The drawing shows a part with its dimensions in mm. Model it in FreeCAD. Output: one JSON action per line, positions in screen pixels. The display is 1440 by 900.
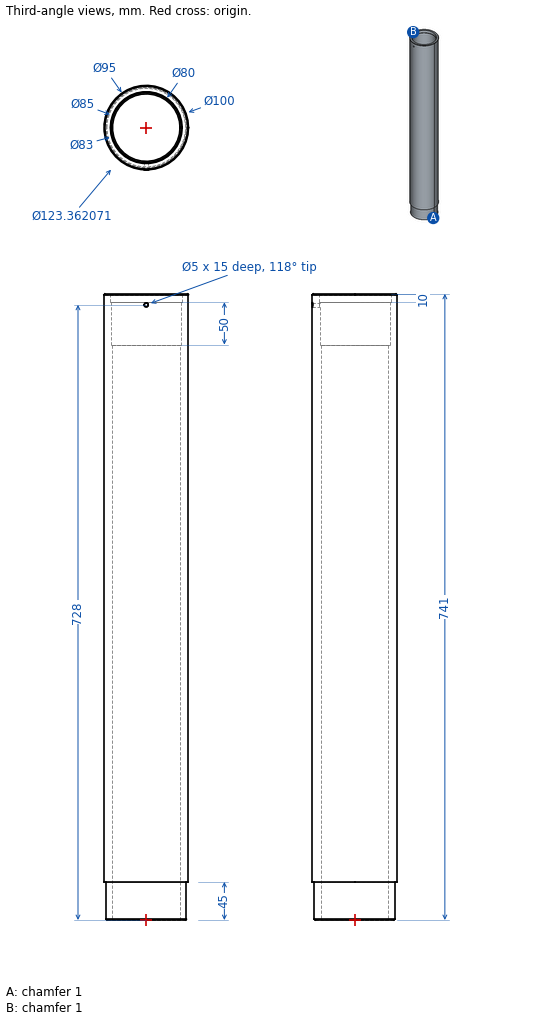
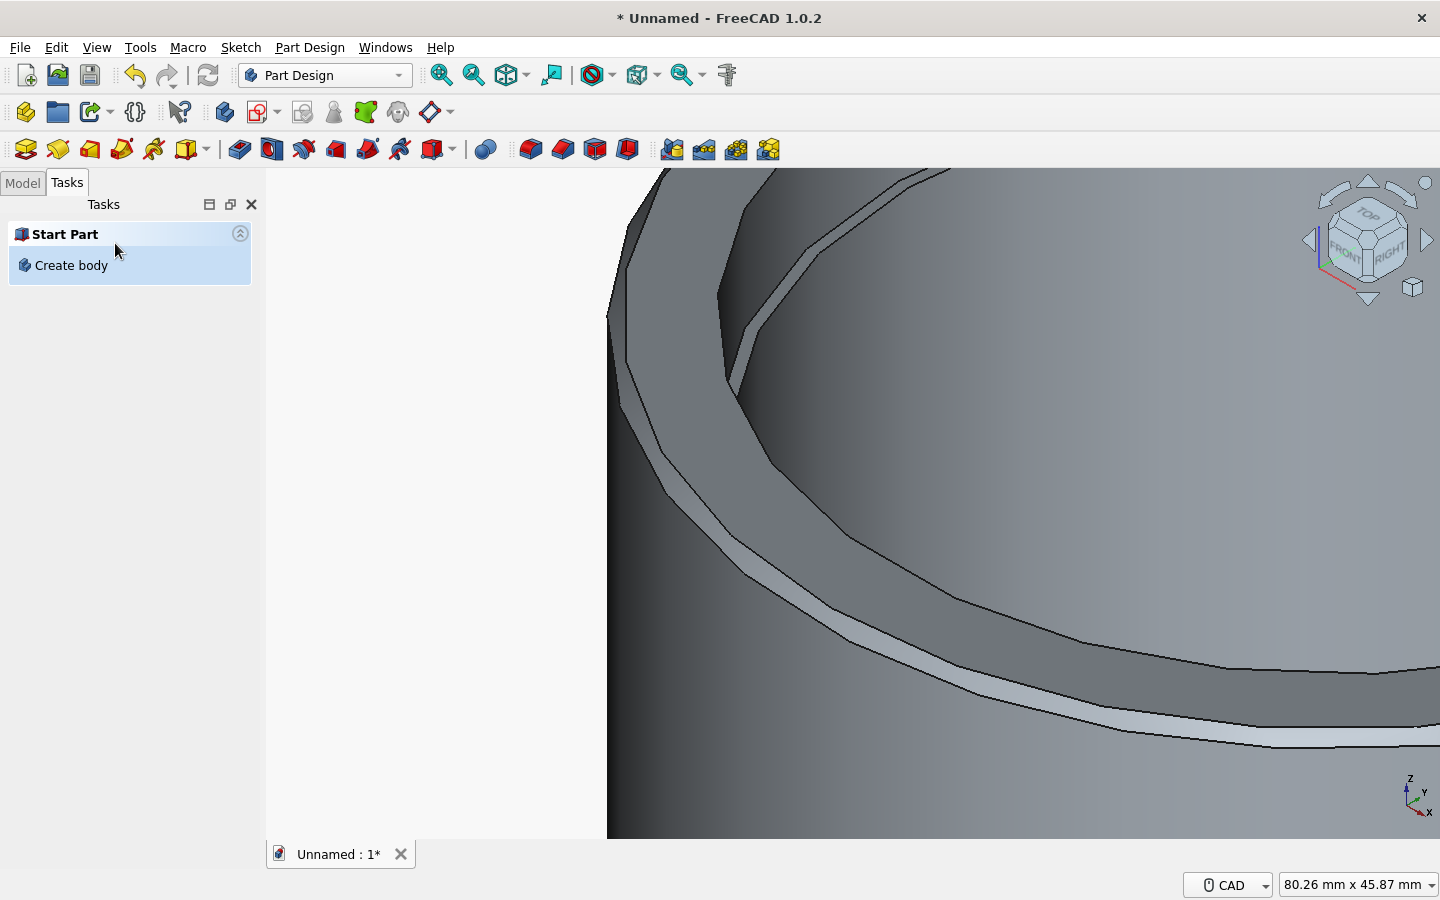
{"action": "left_click", "coordinate": [442, 76]}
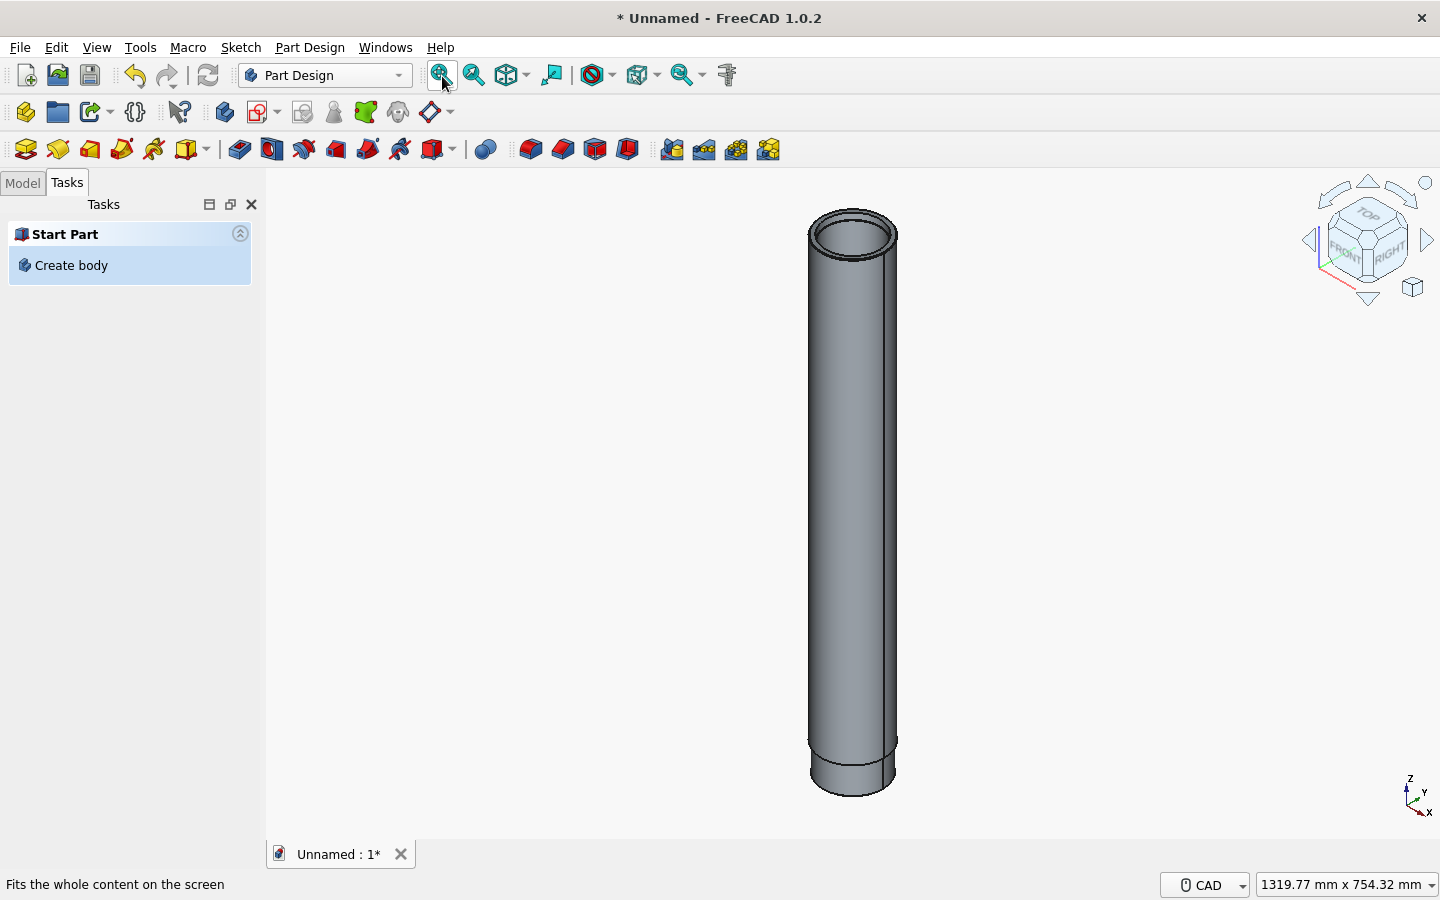
{"action": "left_click", "coordinate": [23, 182]}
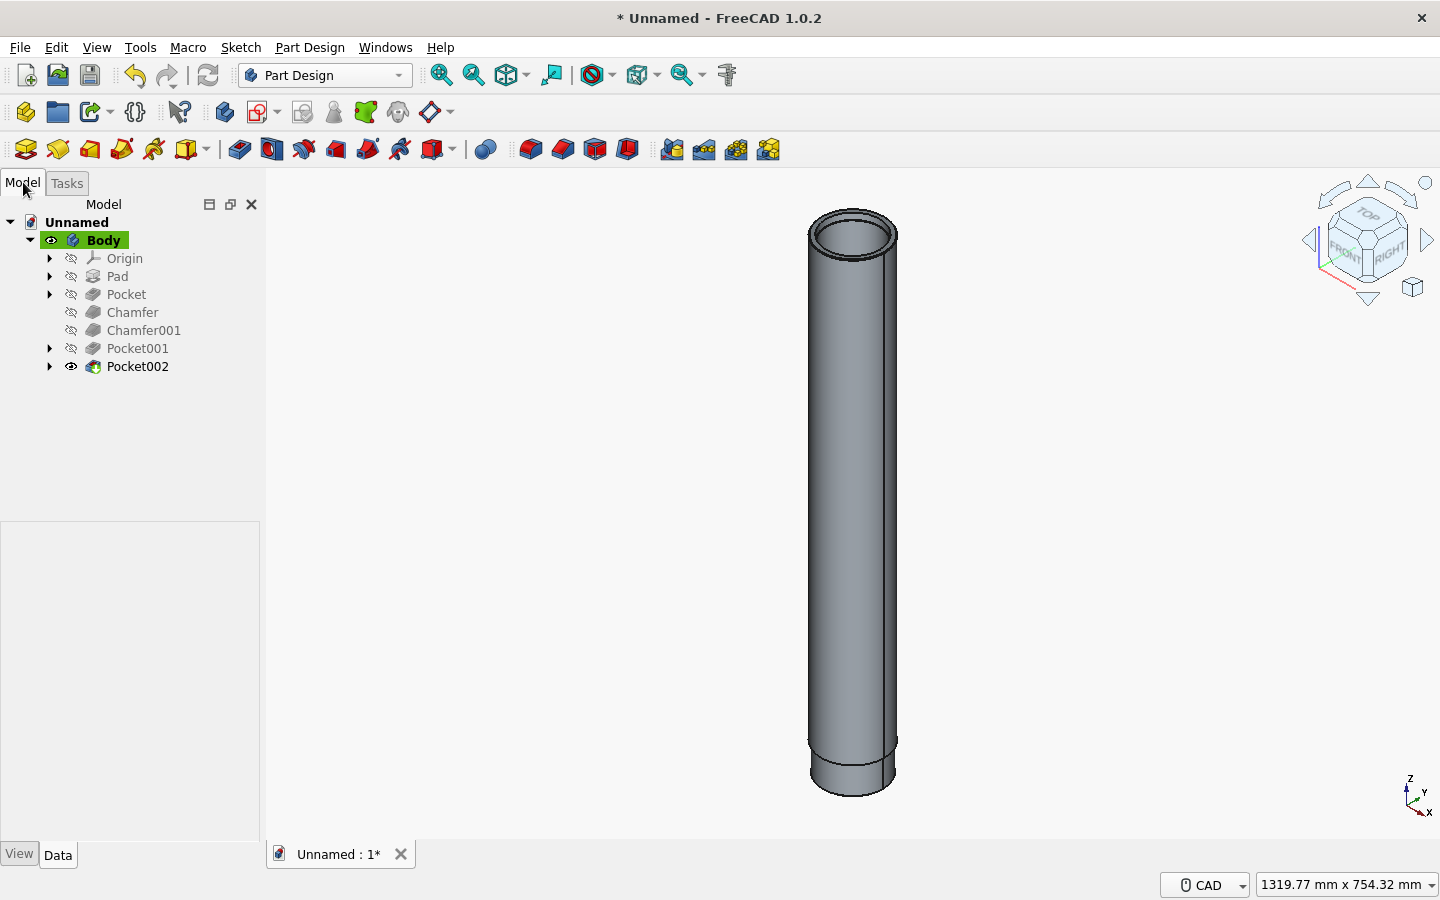
{"action": "left_click", "coordinate": [50, 258]}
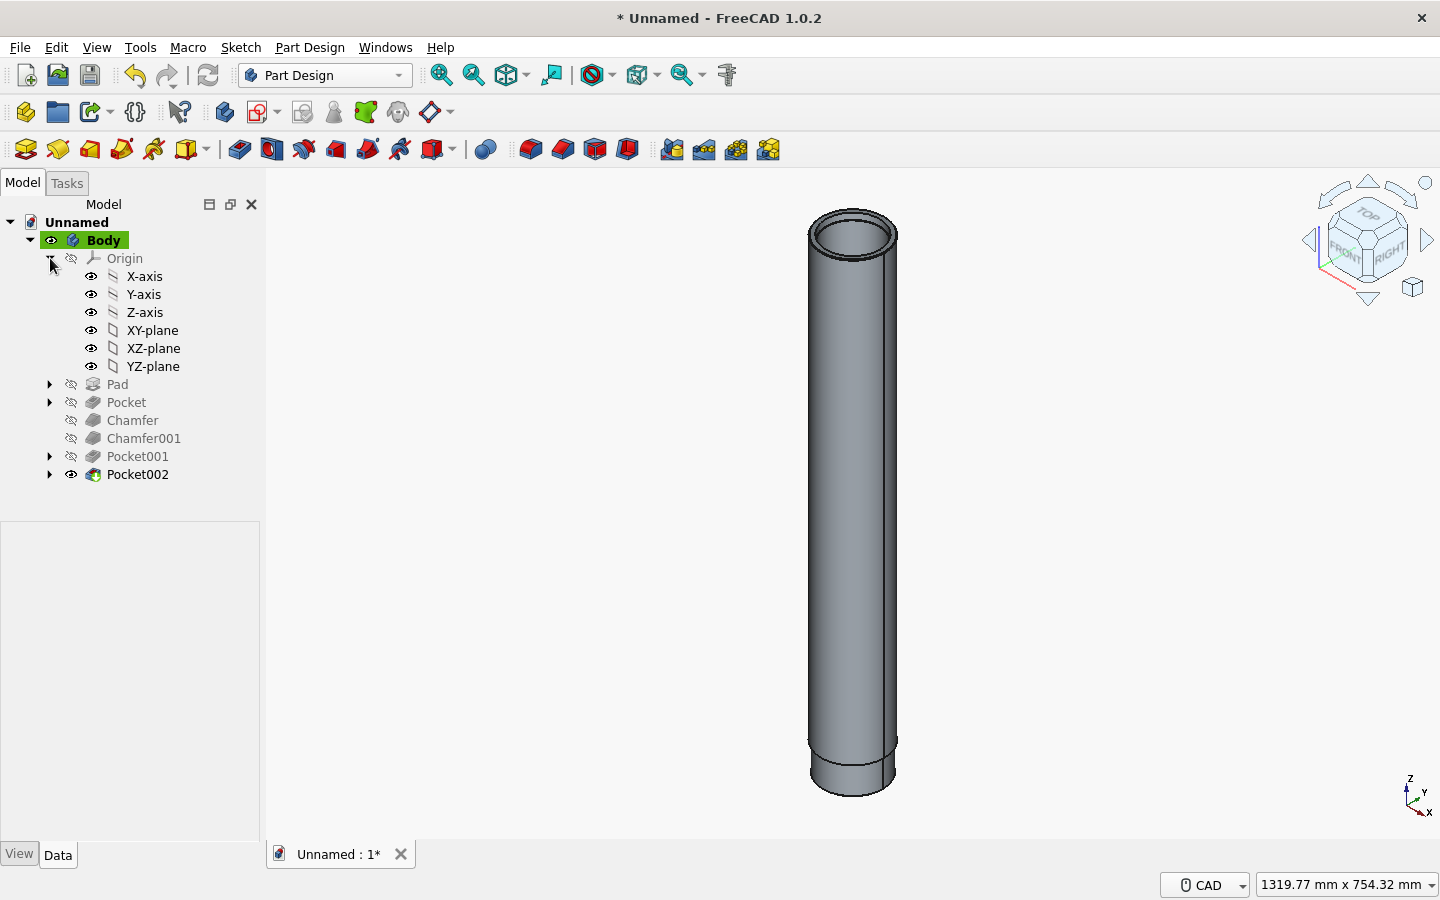
{"action": "left_click", "coordinate": [136, 348]}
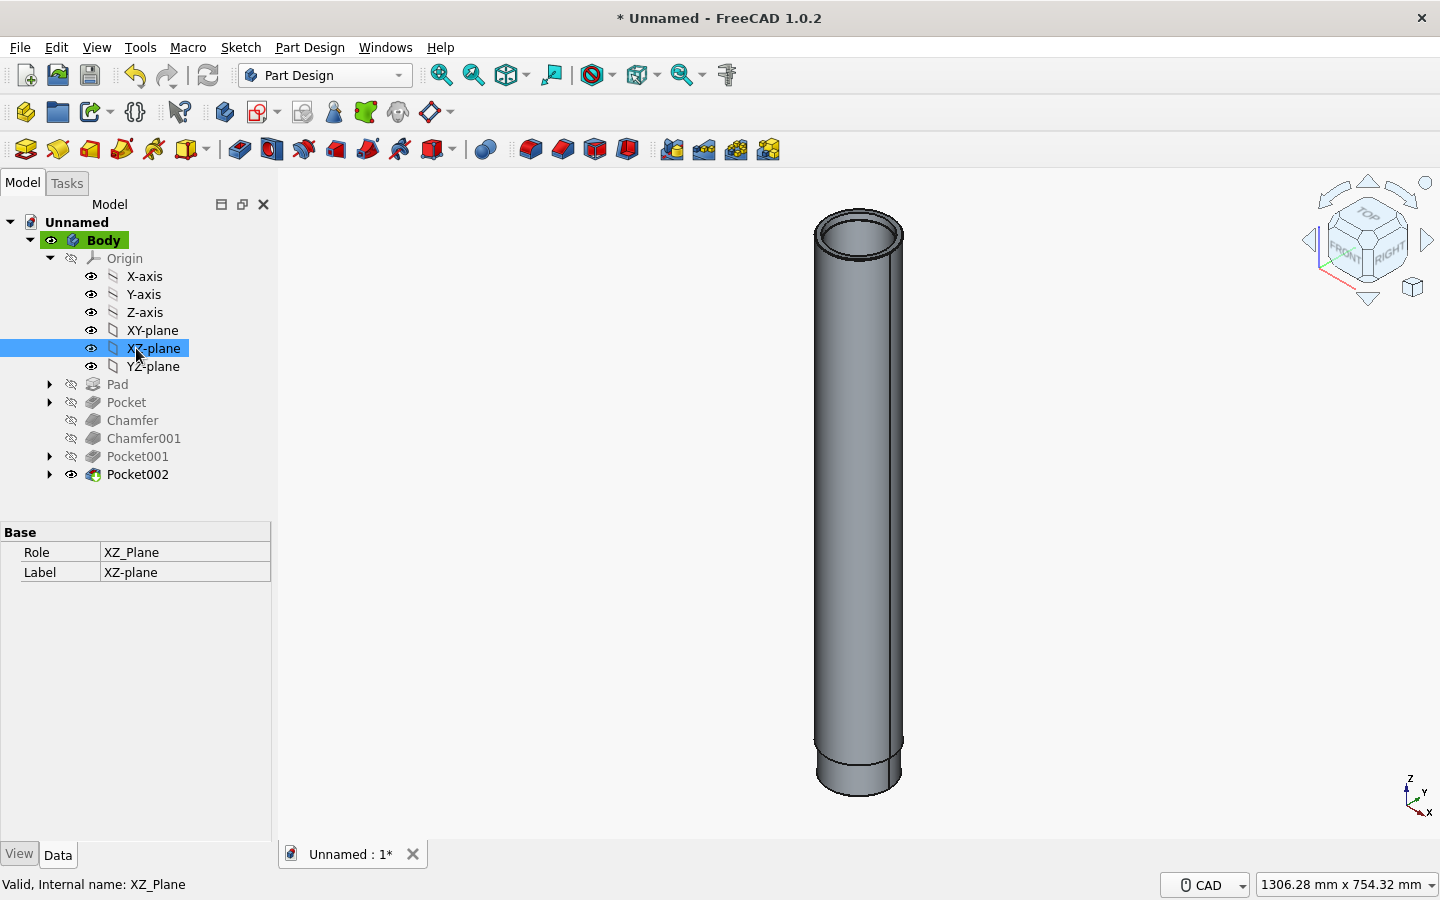
{"action": "left_click", "coordinate": [430, 112]}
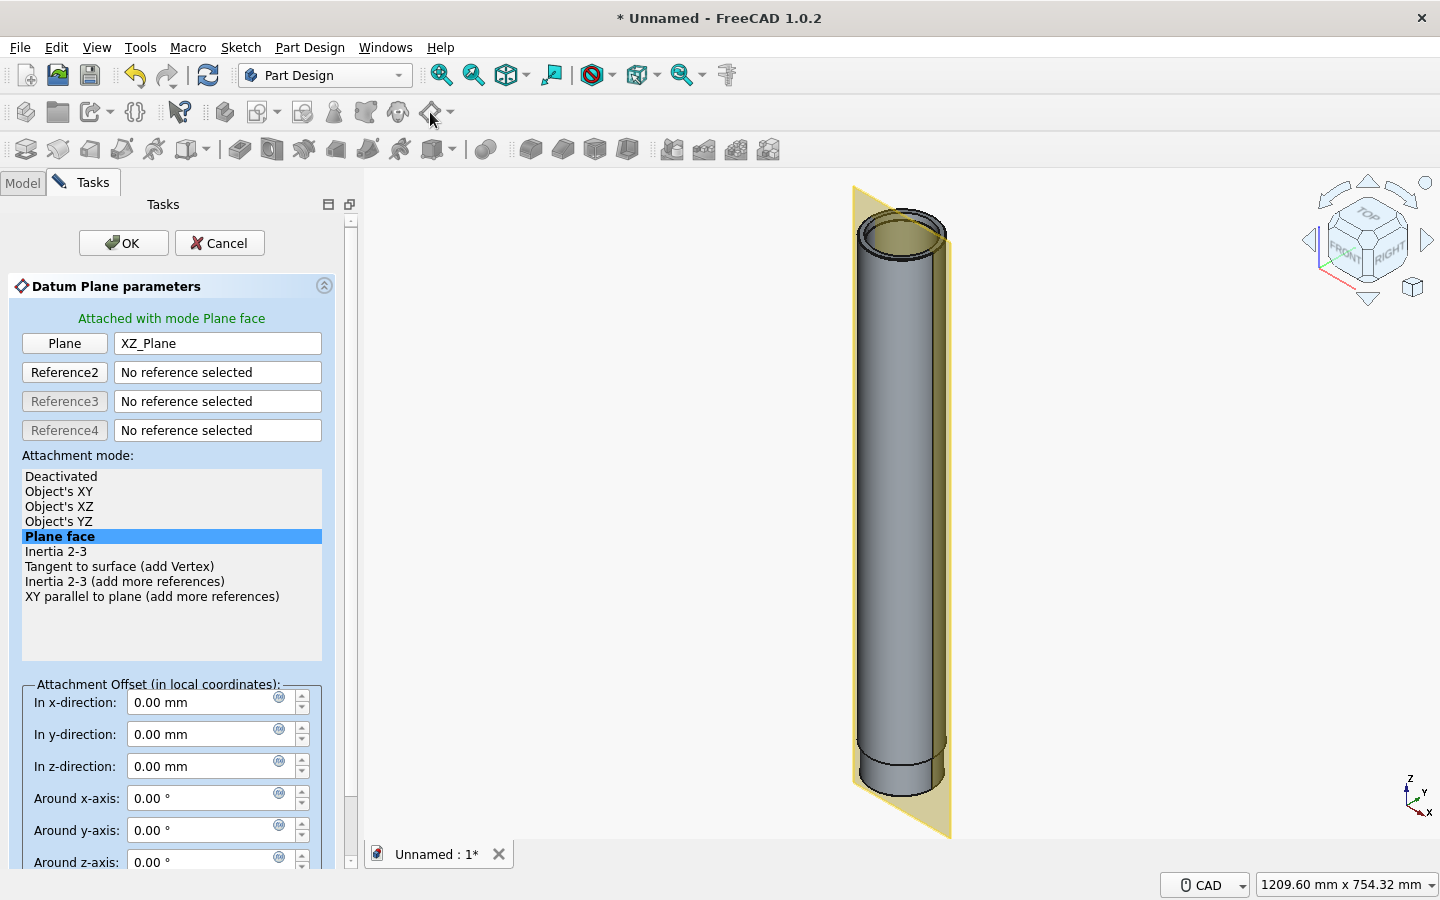
{"action": "triple_click", "coordinate": [210, 766]}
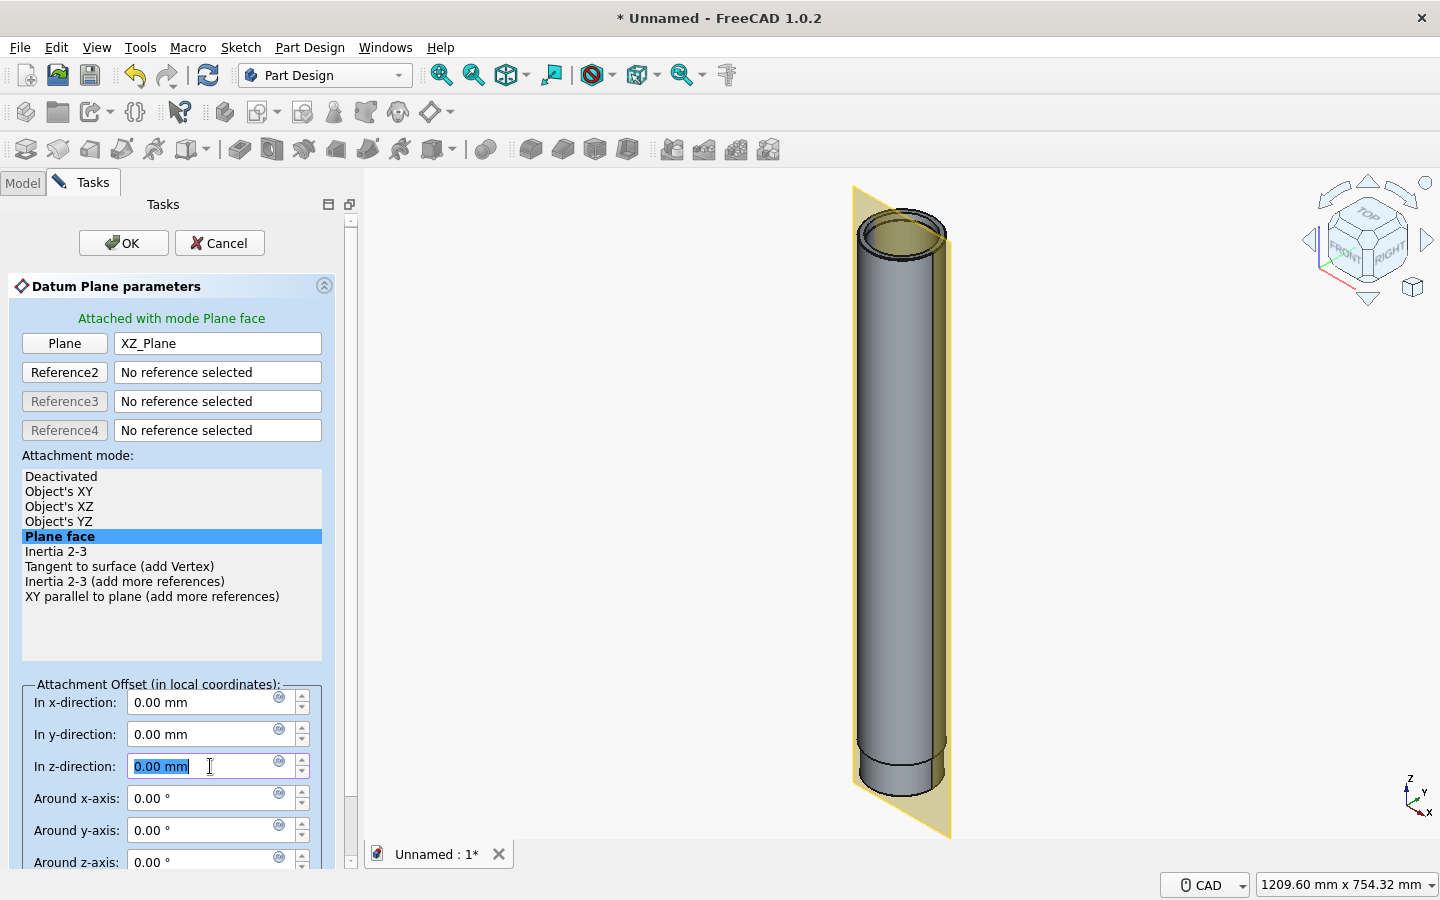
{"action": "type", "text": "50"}
{"action": "key", "text": "Tab"}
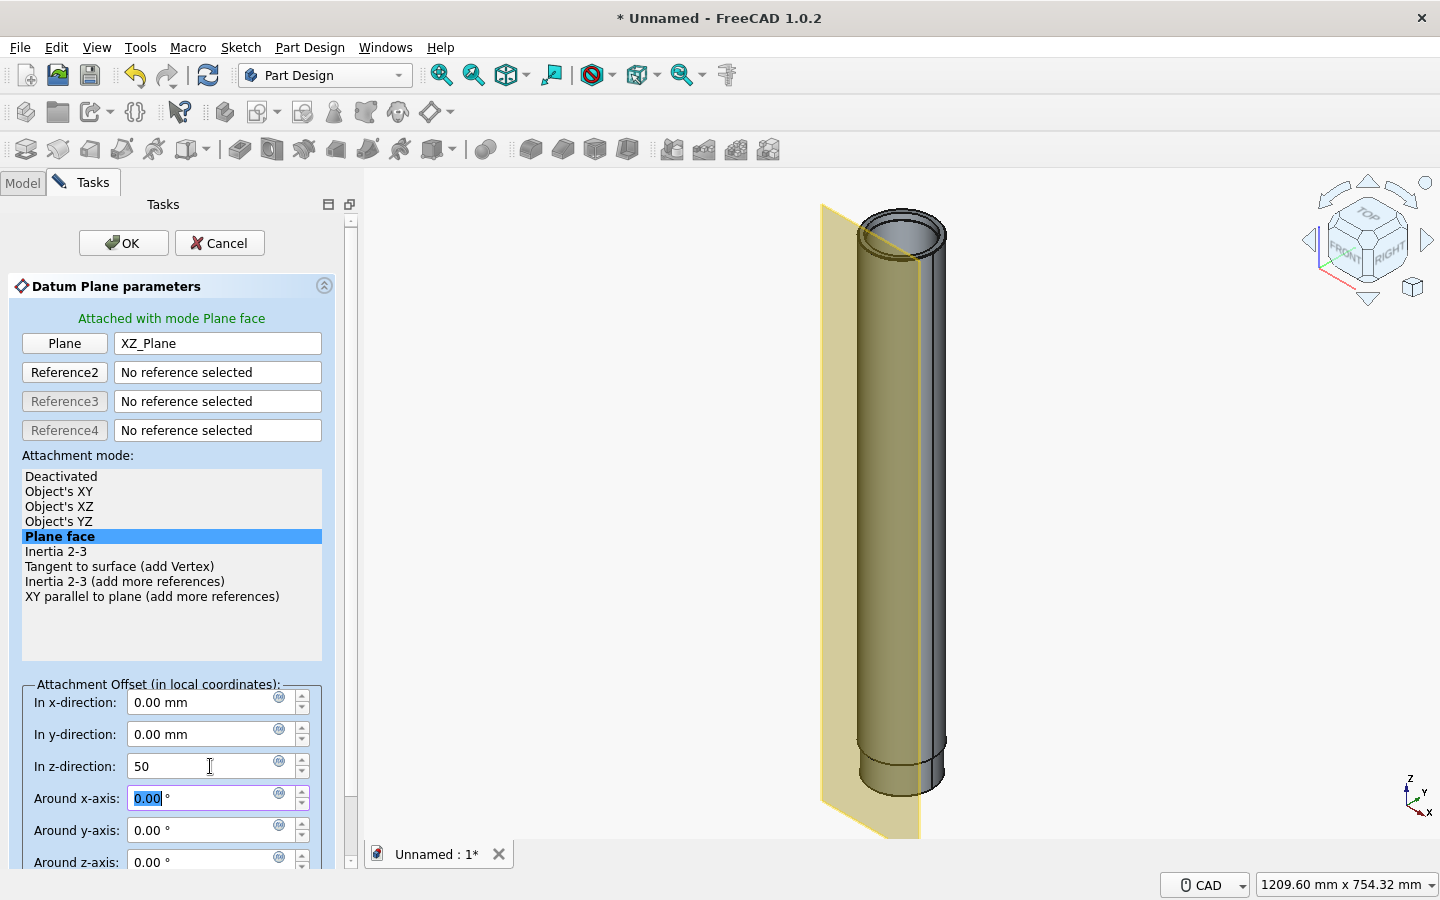
{"action": "left_click", "coordinate": [124, 243]}